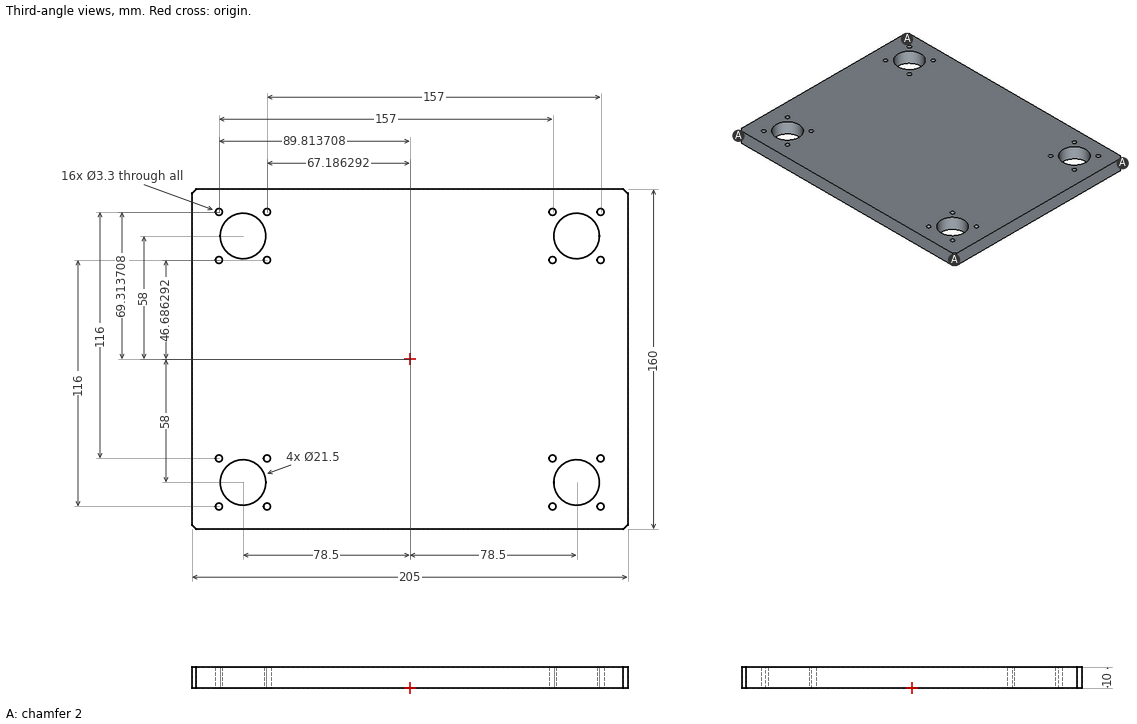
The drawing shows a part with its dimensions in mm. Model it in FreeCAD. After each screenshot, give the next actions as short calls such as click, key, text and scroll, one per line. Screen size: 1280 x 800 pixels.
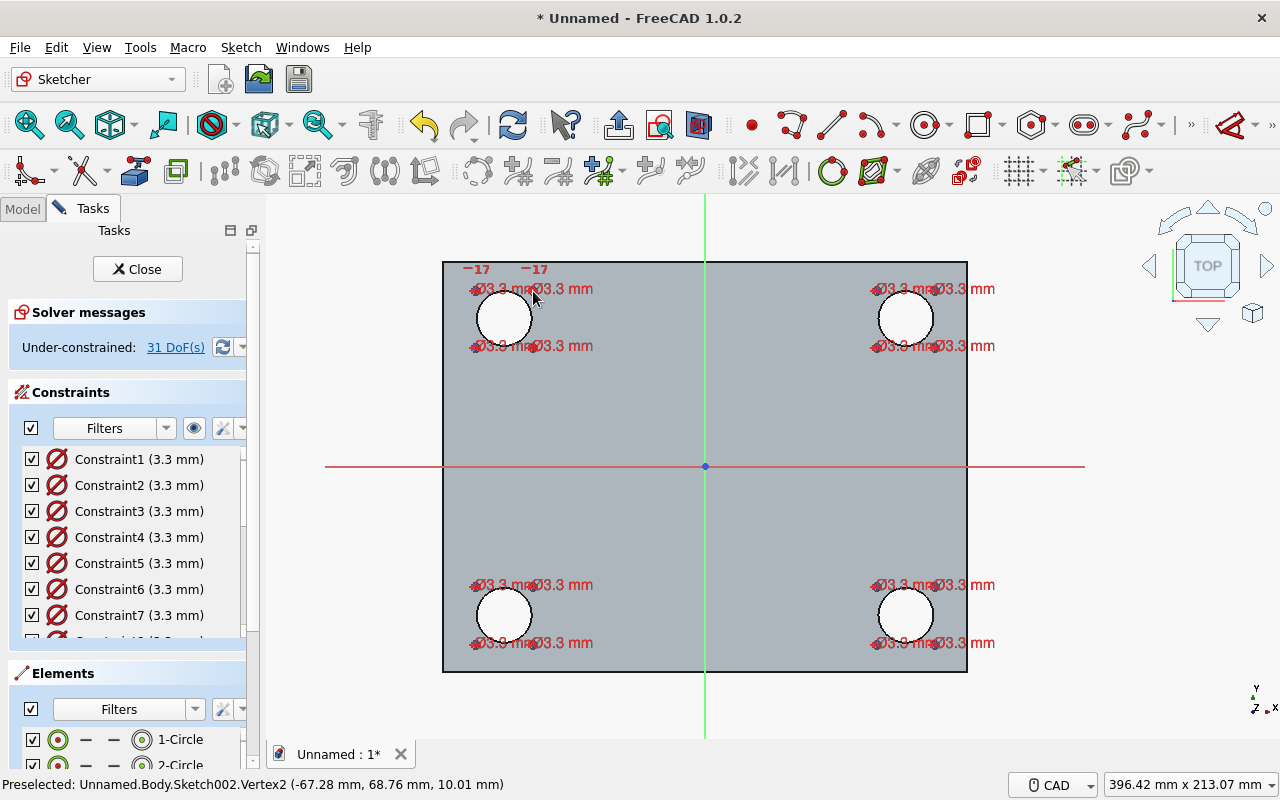
click(533, 291)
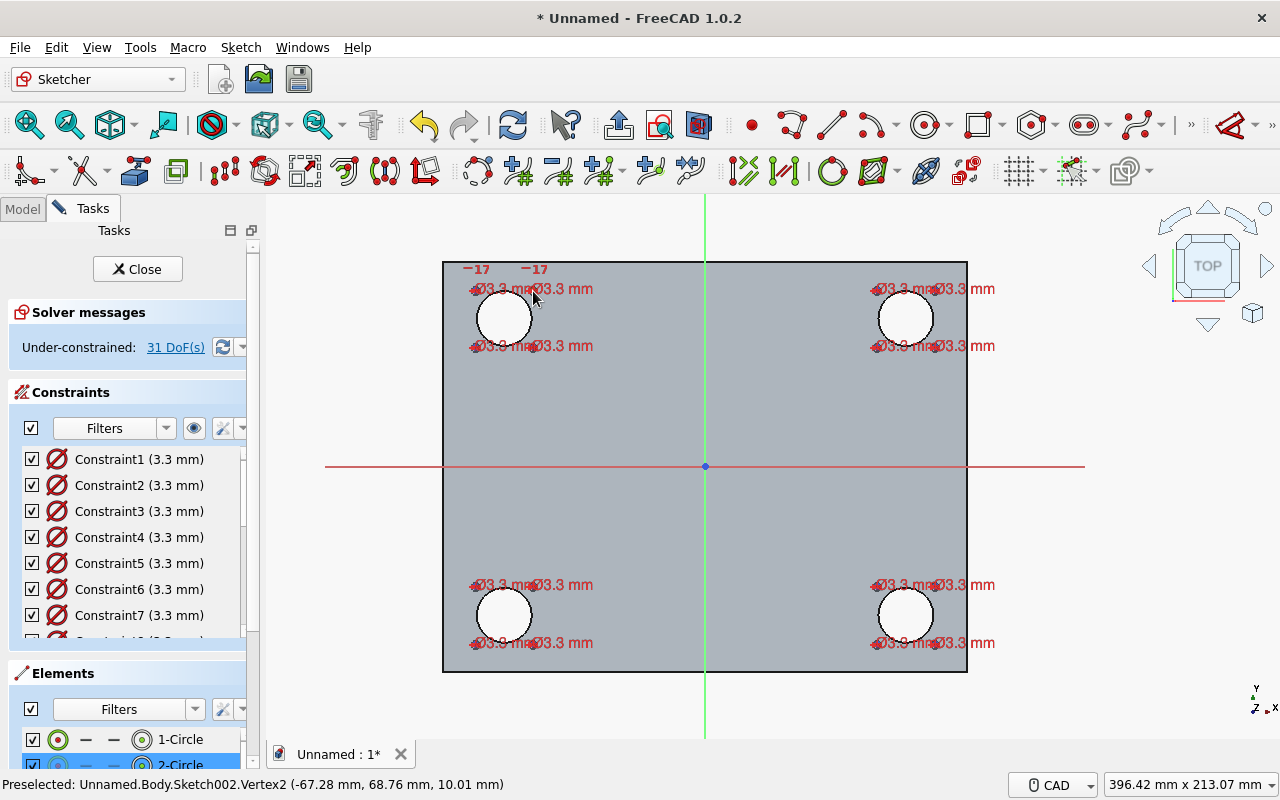
click(533, 348)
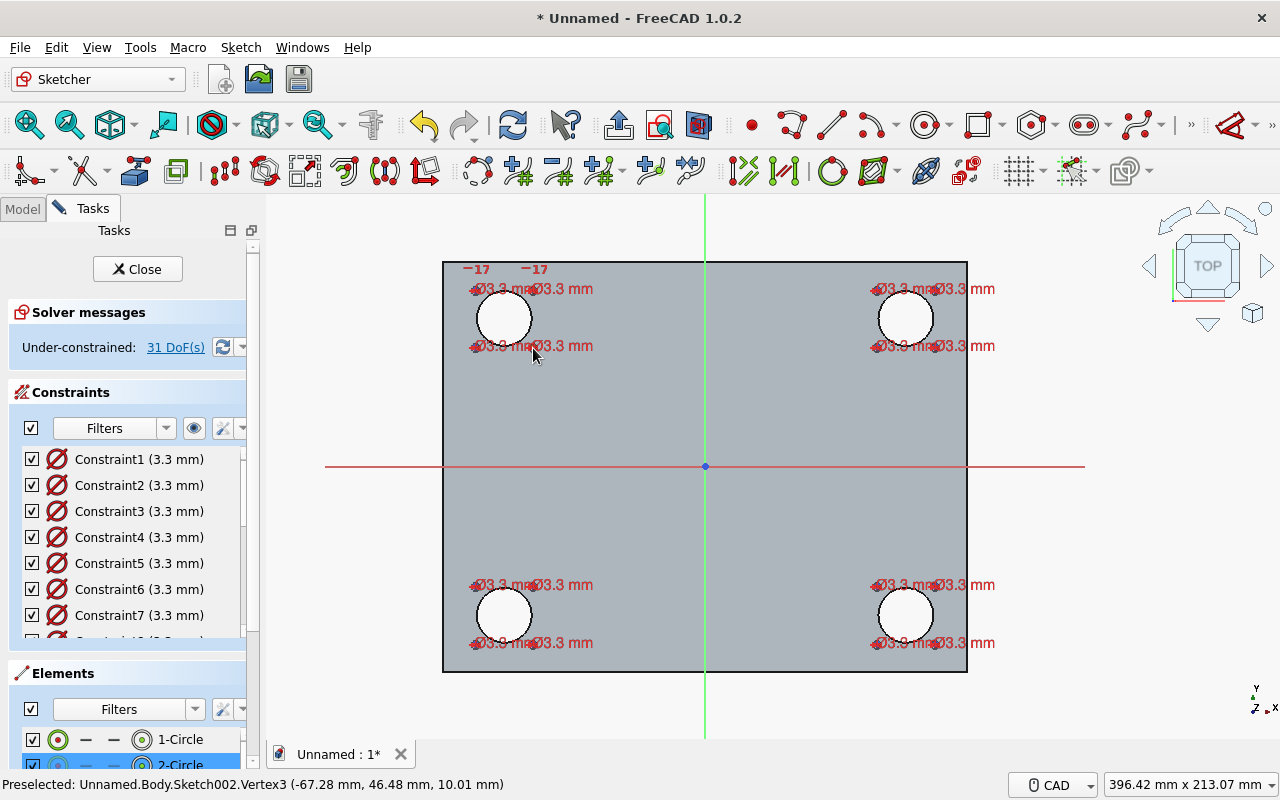
key(v)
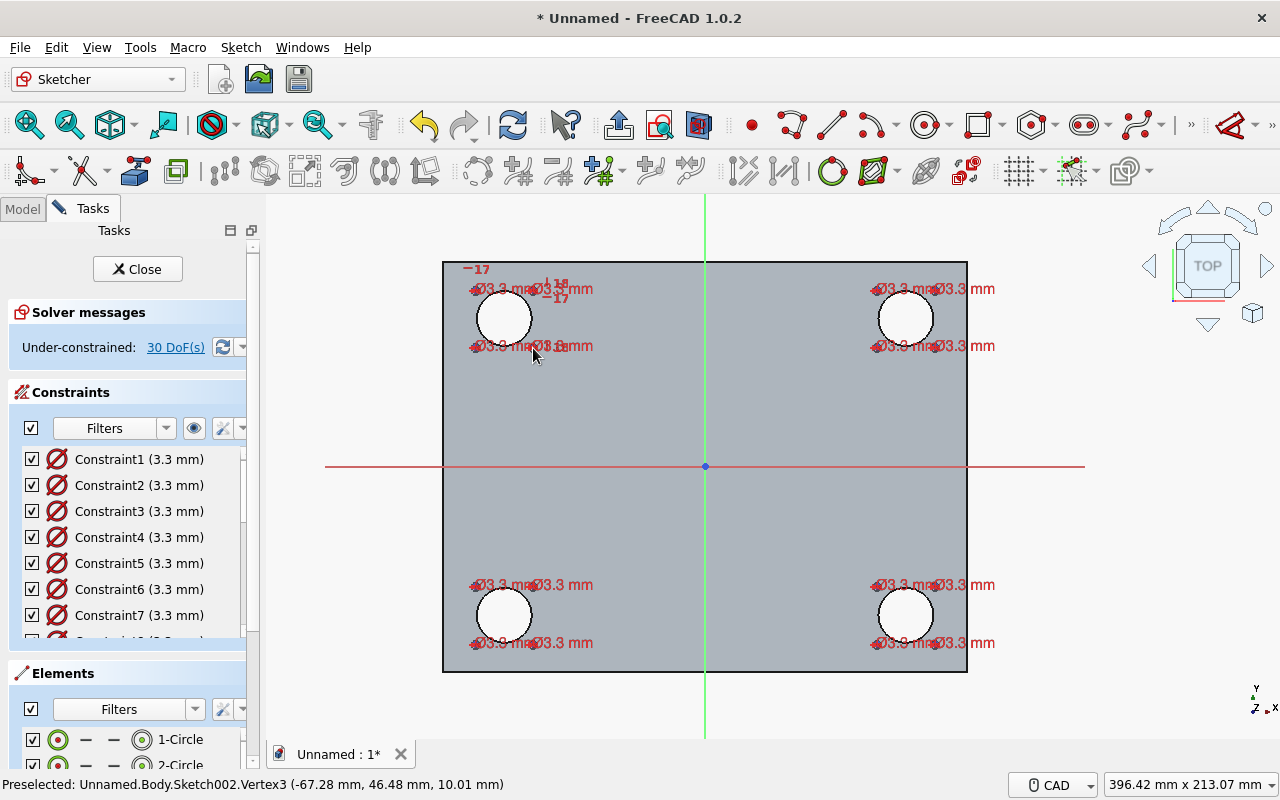
click(476, 291)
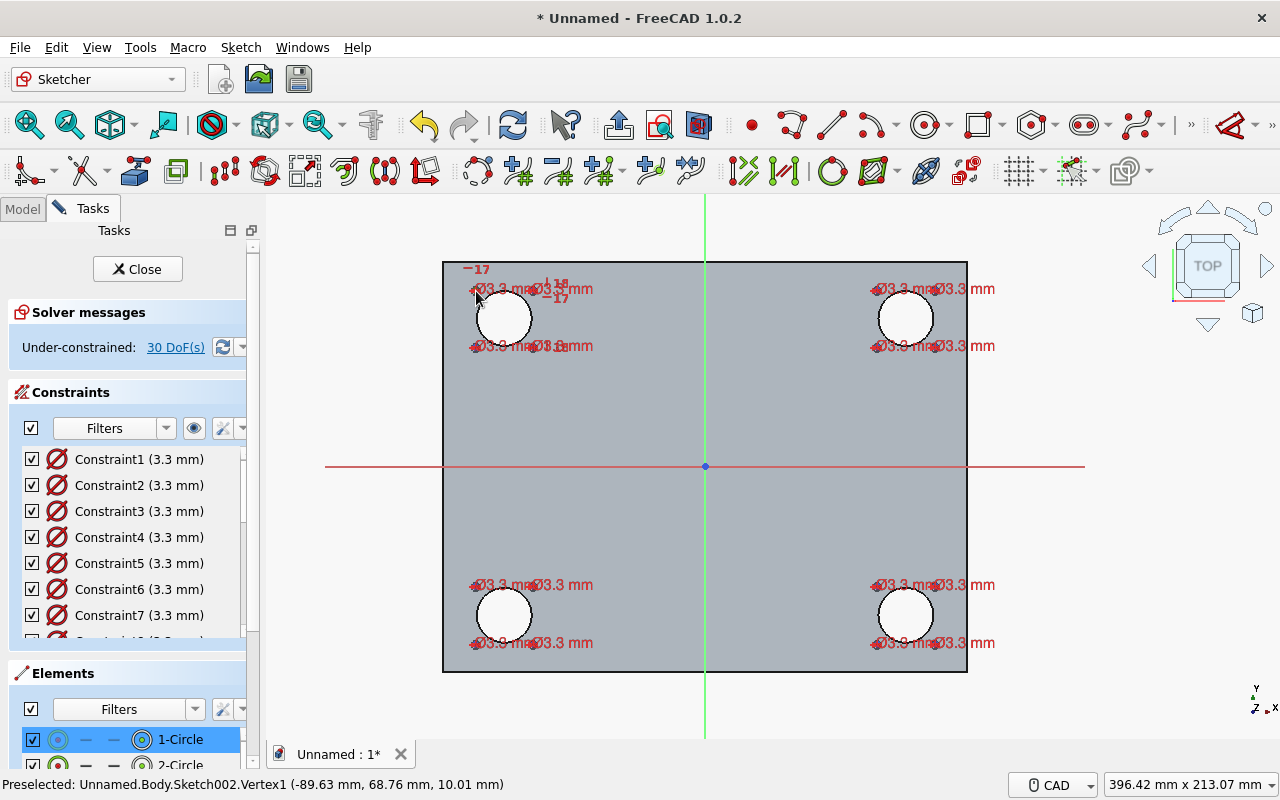
click(476, 348)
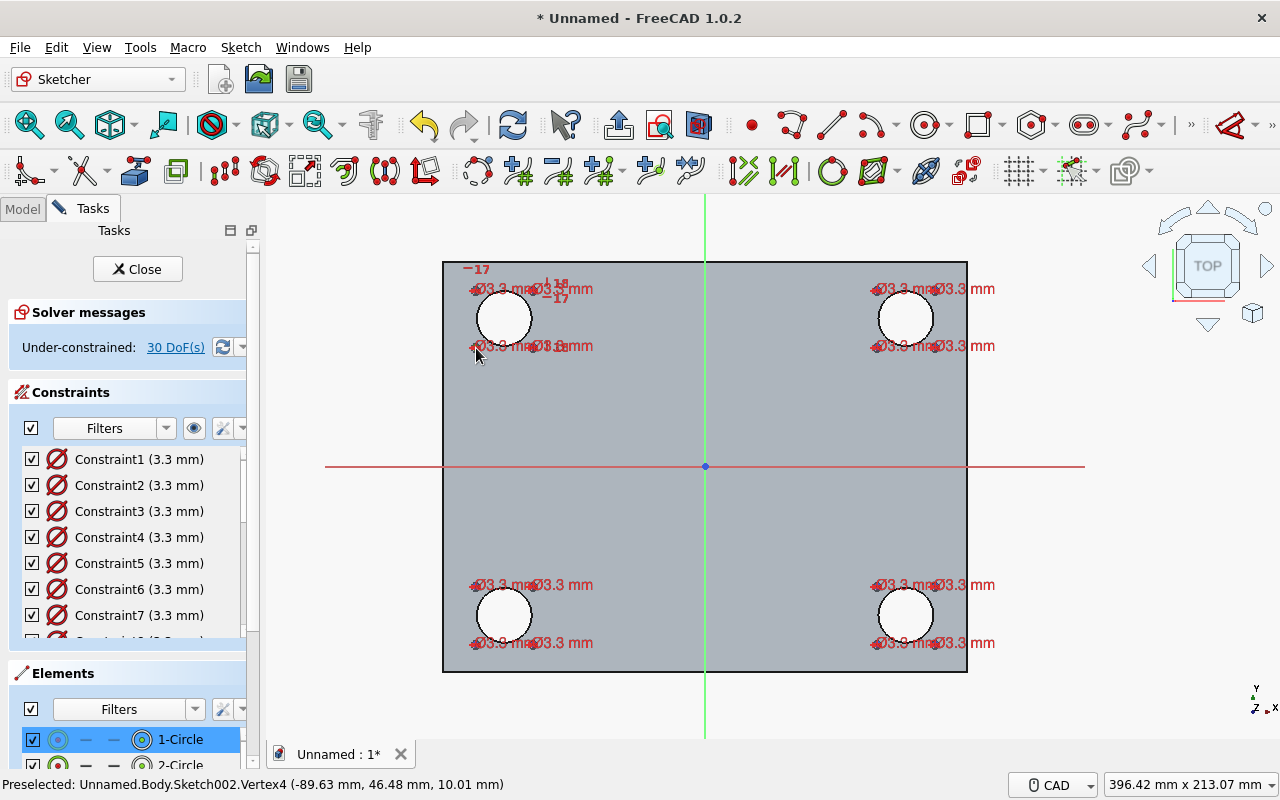
key(v)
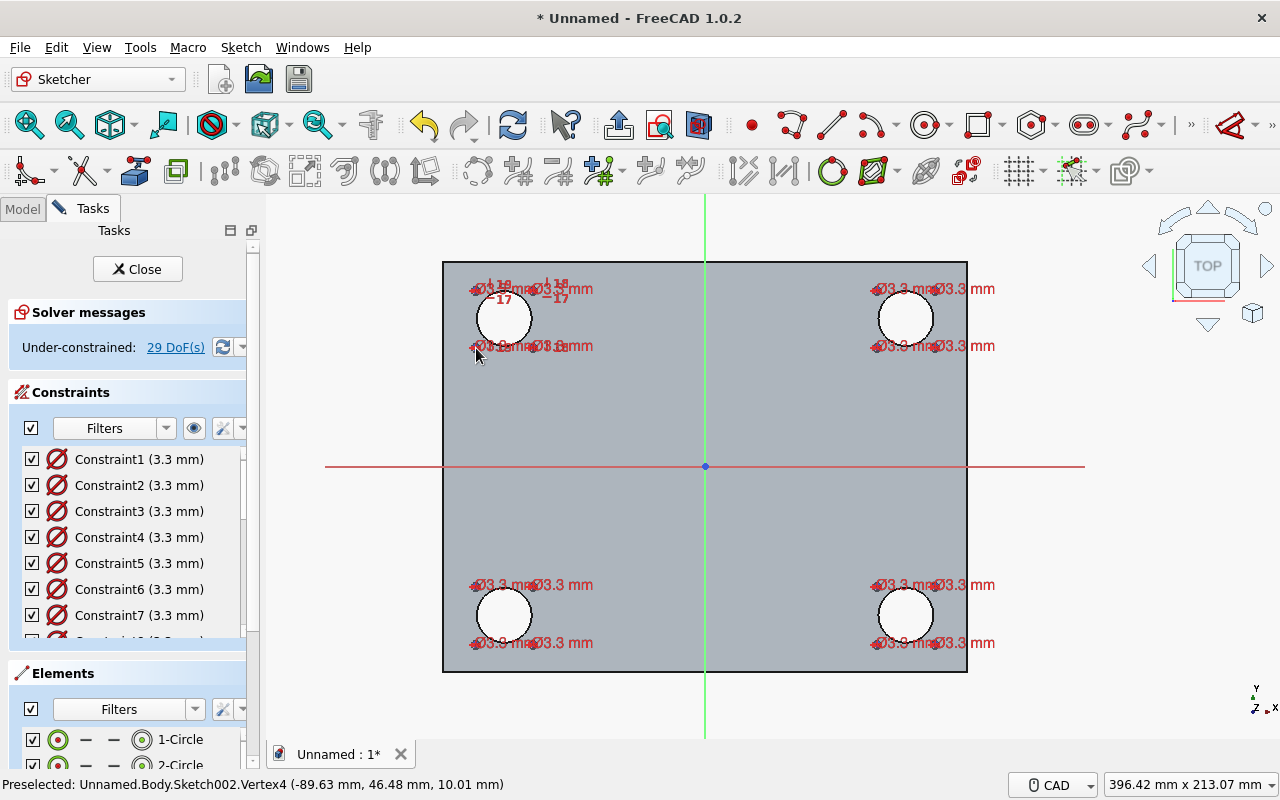
click(533, 348)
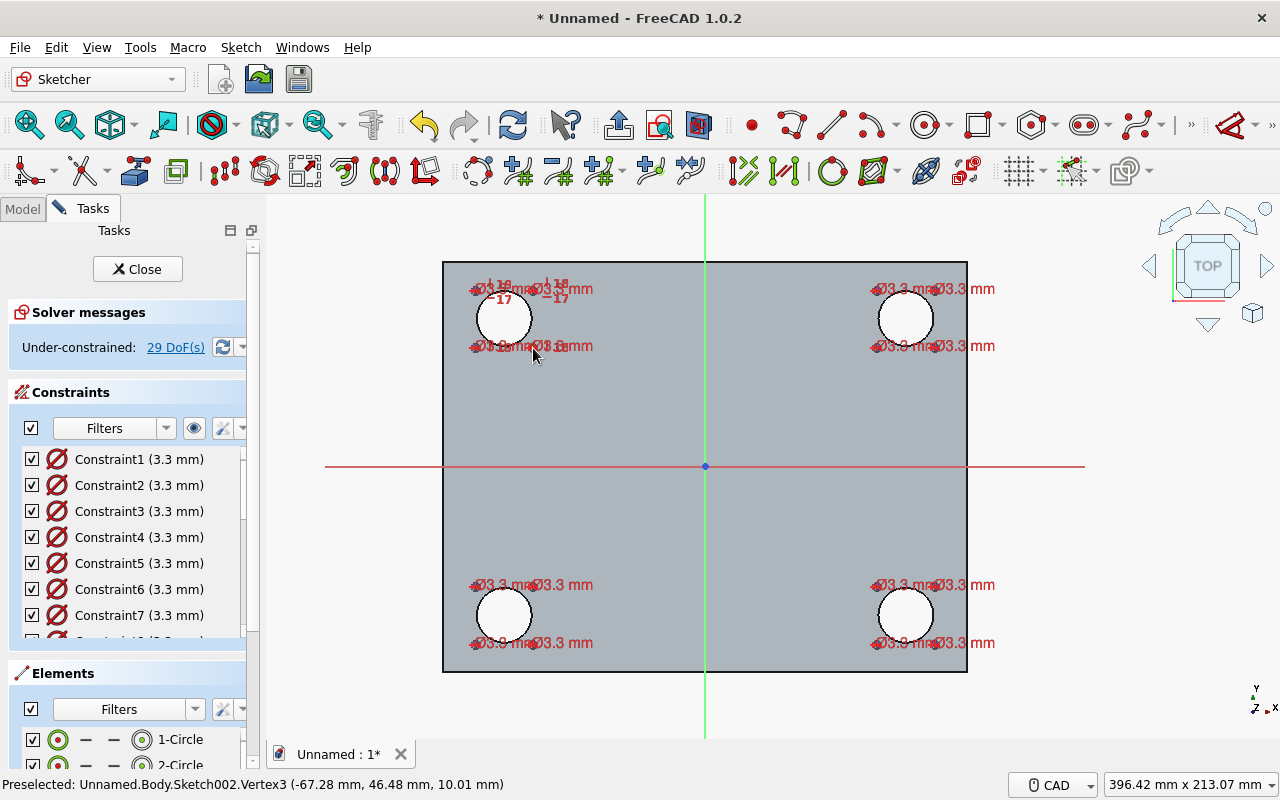
click(476, 348)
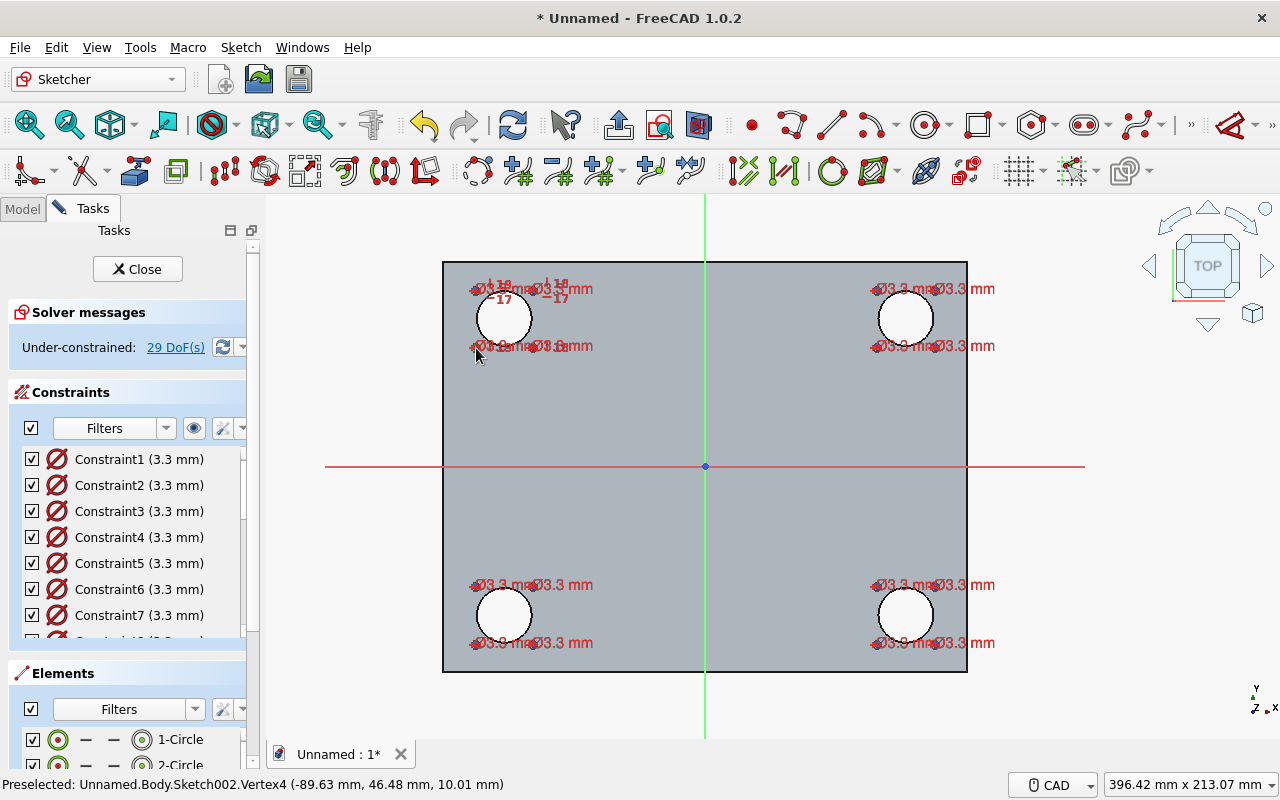
key(h)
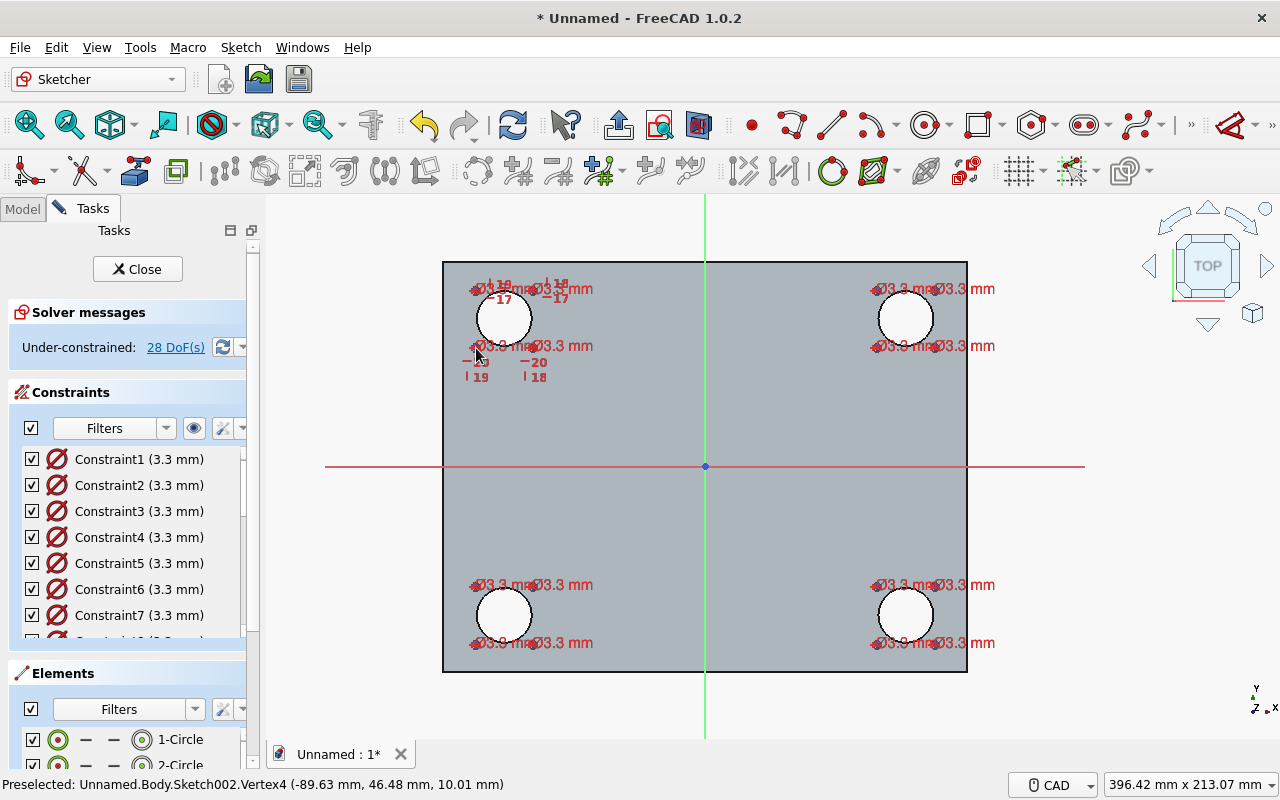
click(533, 291)